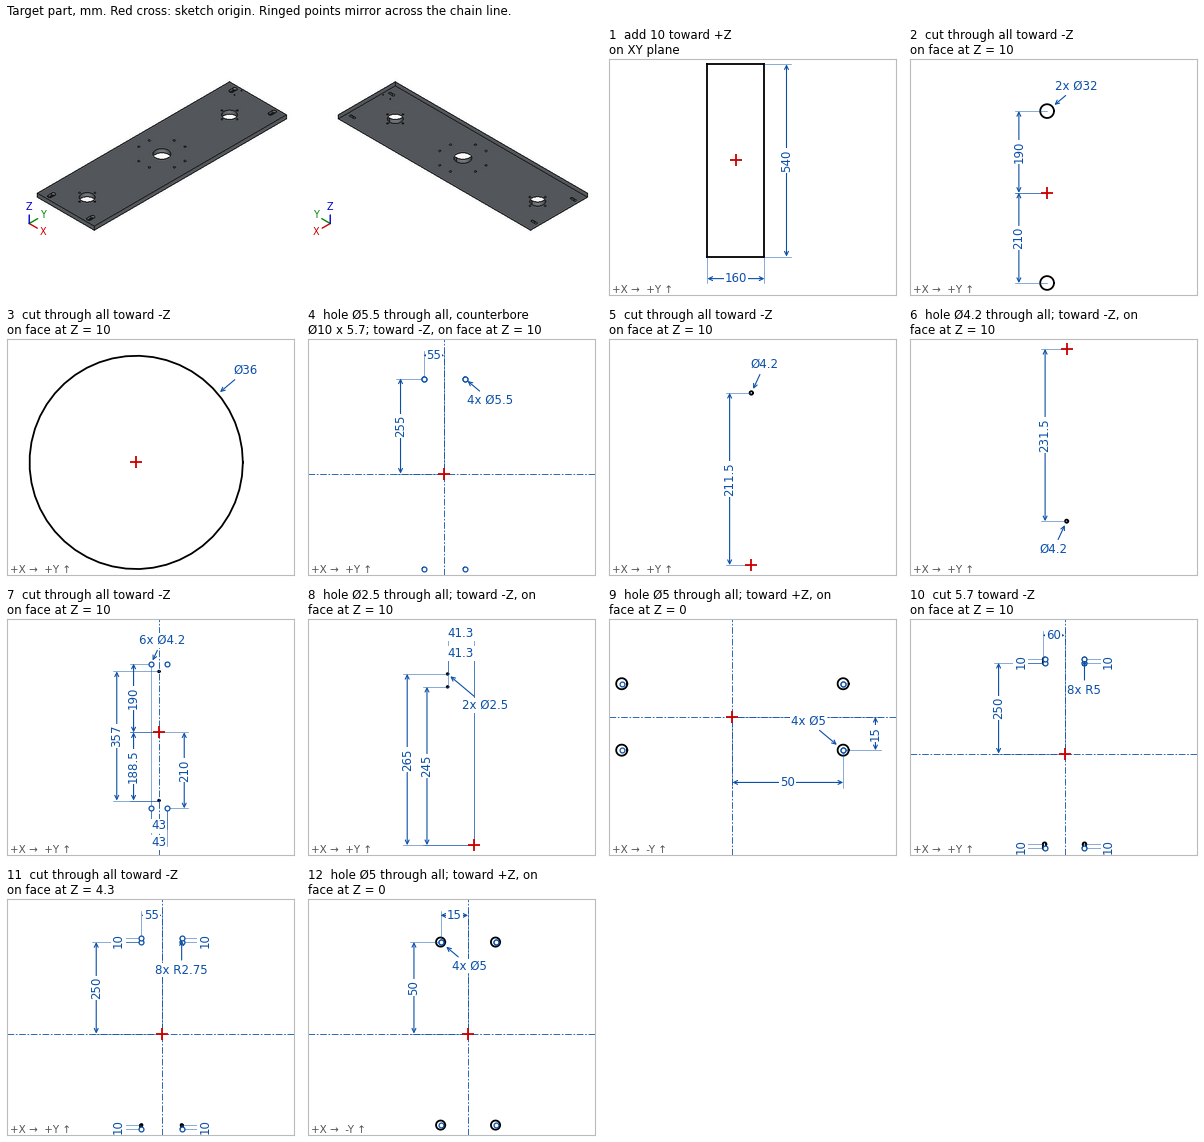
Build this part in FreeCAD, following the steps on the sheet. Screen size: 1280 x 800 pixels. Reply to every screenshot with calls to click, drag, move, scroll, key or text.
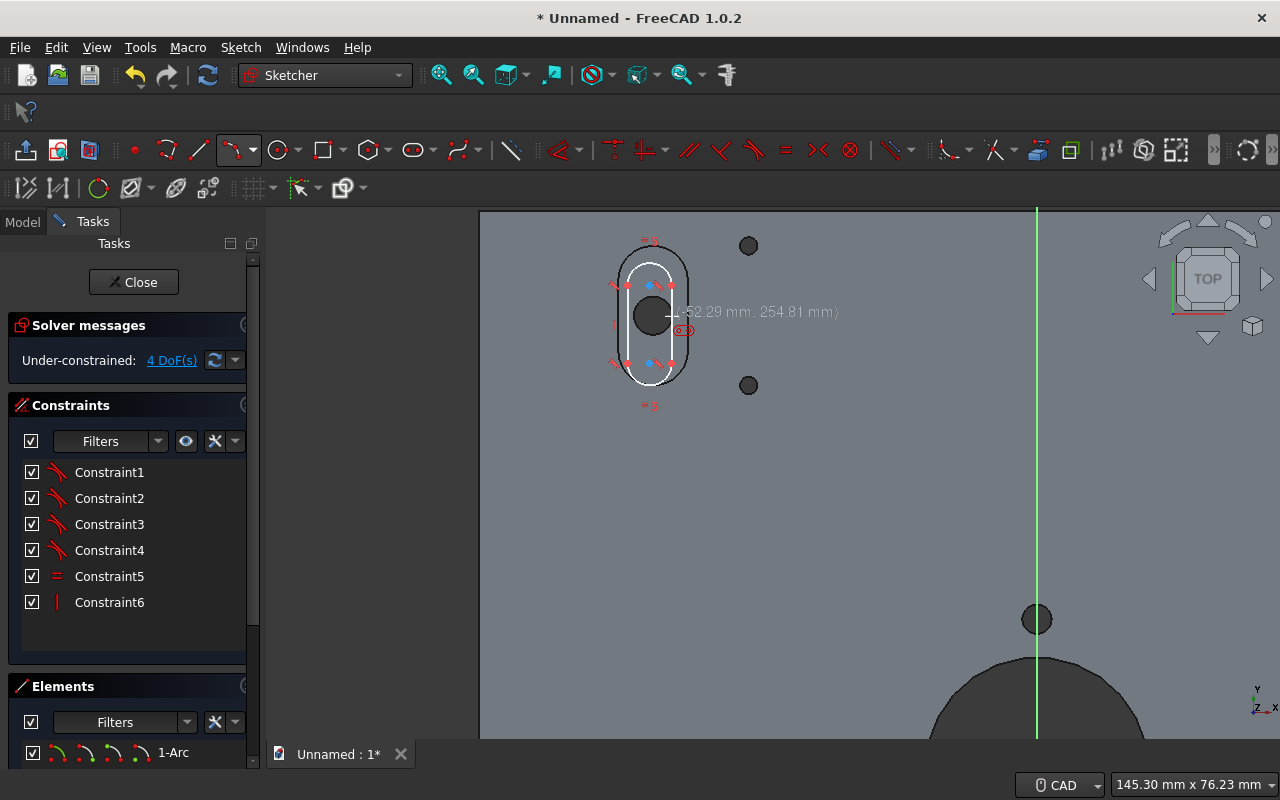
scroll(671, 311, down, 12)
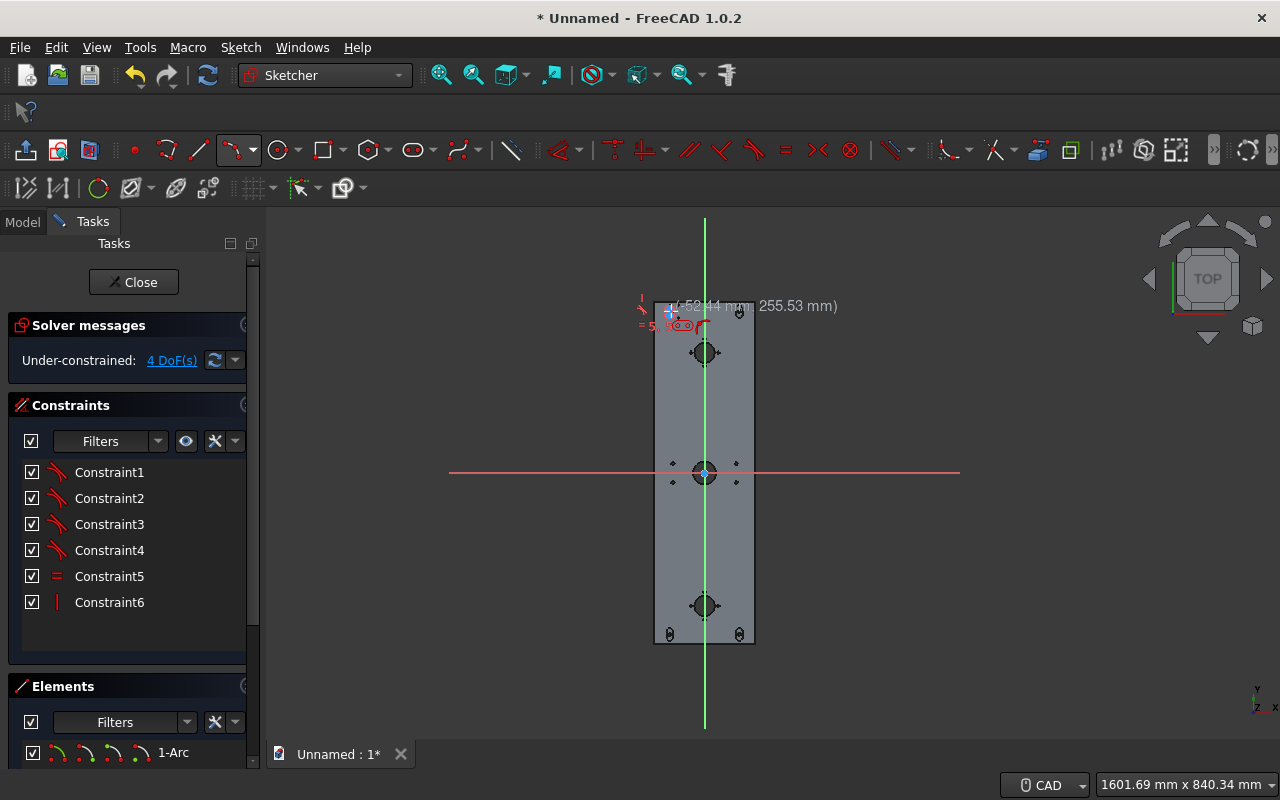
scroll(739, 315, up, 13)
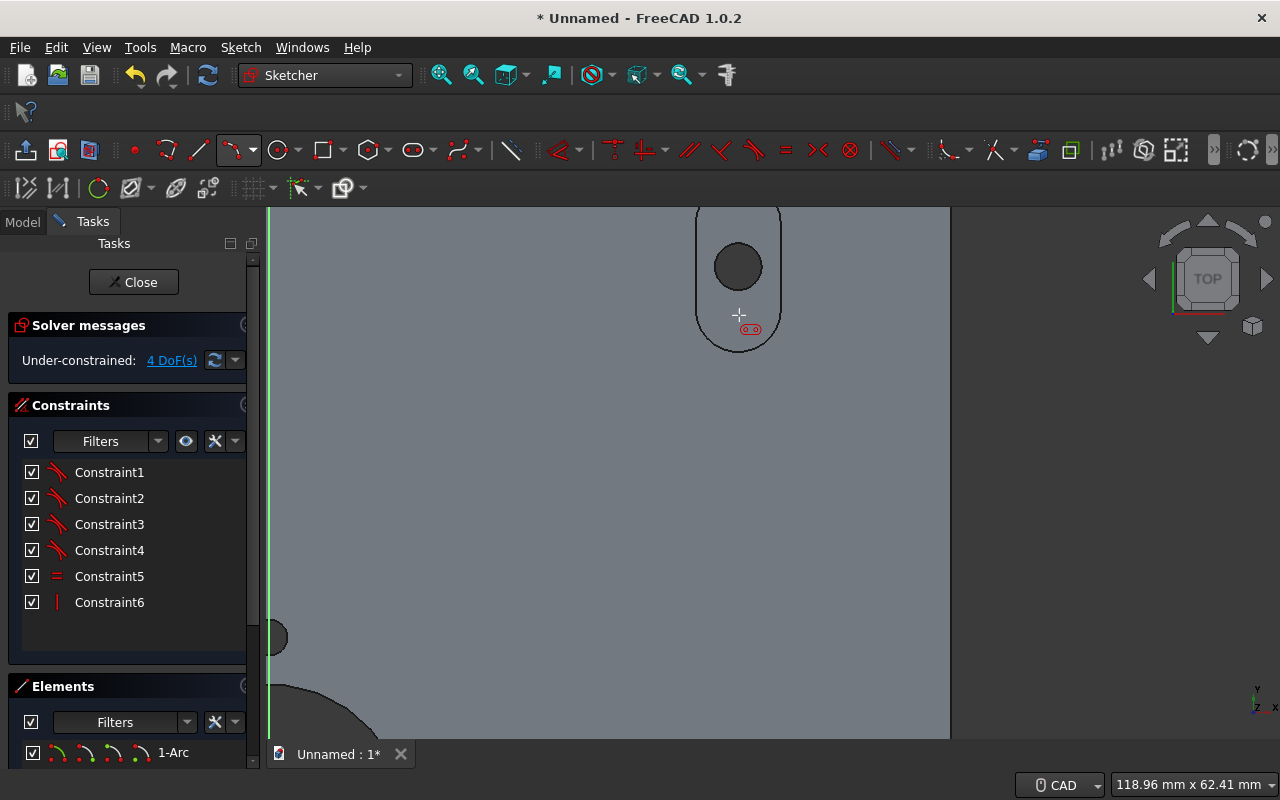
scroll(739, 315, down, 13)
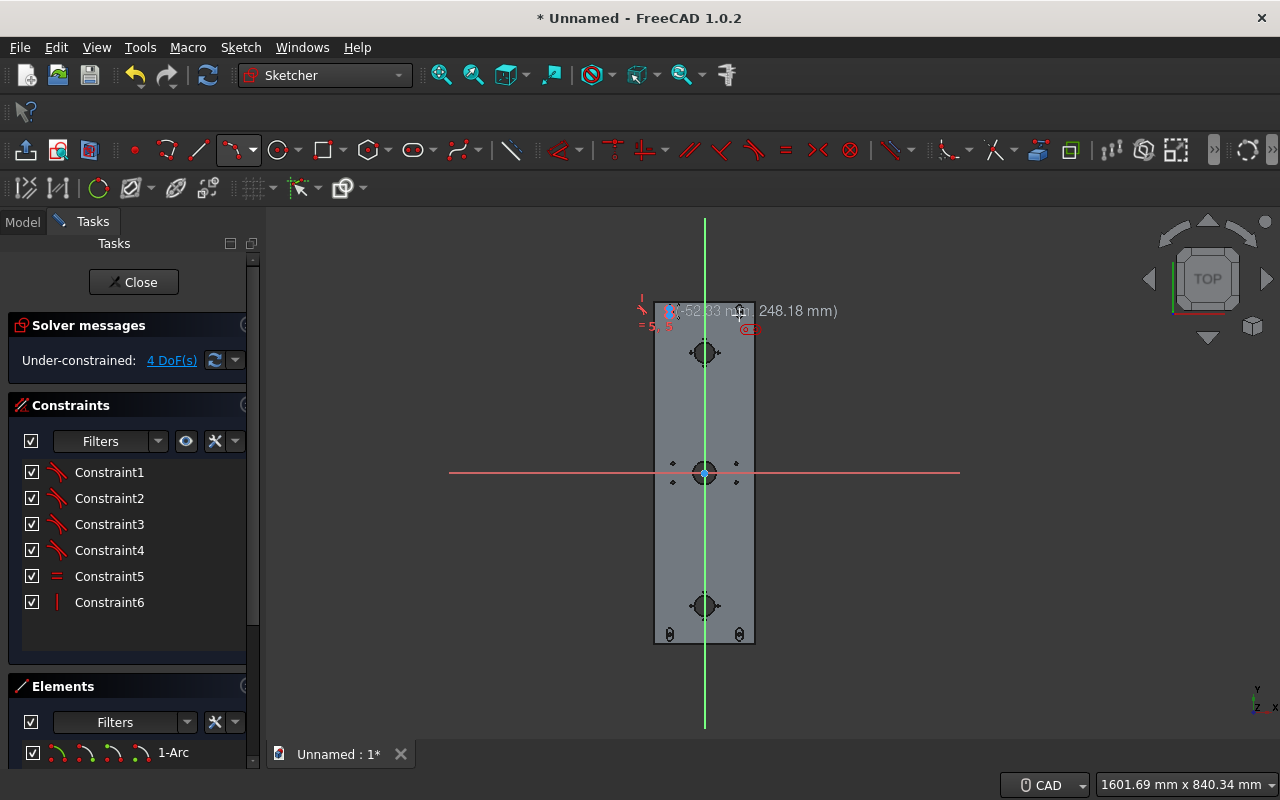
click(739, 315)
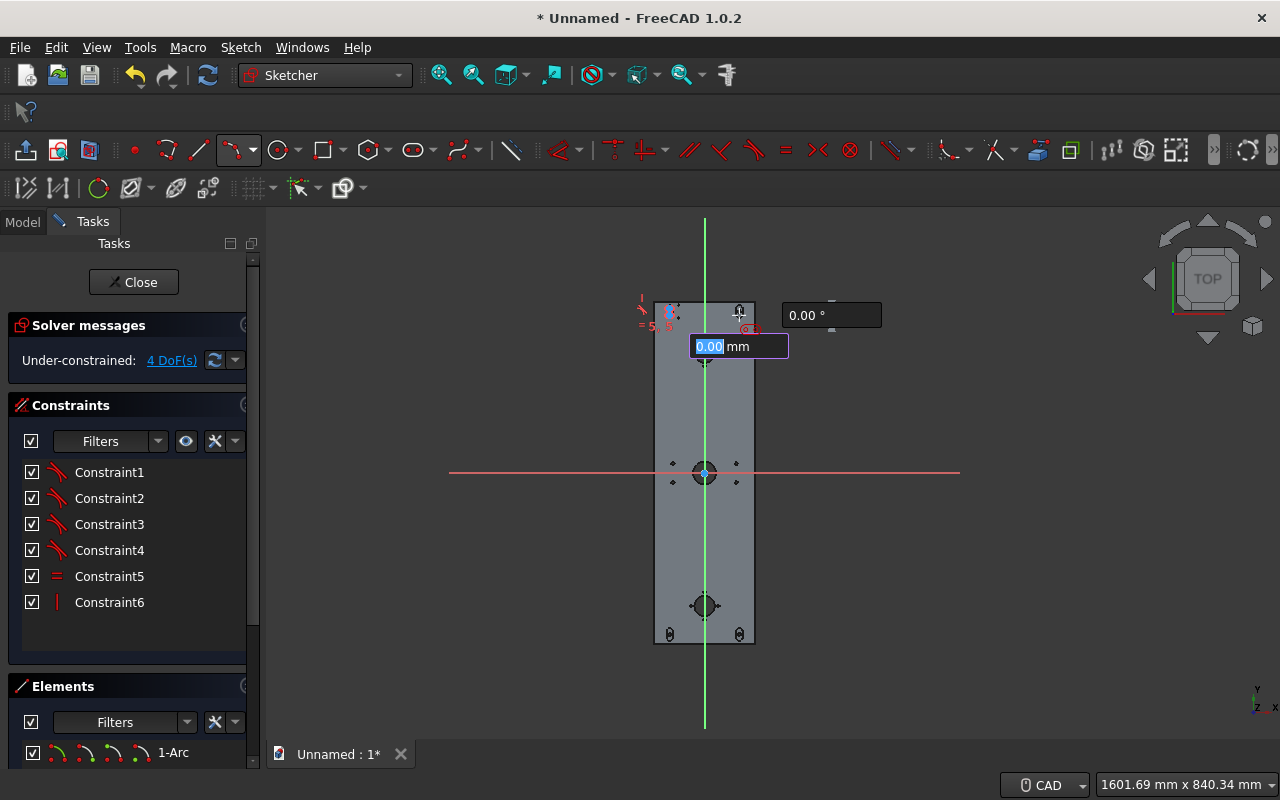
scroll(739, 308, up, 5)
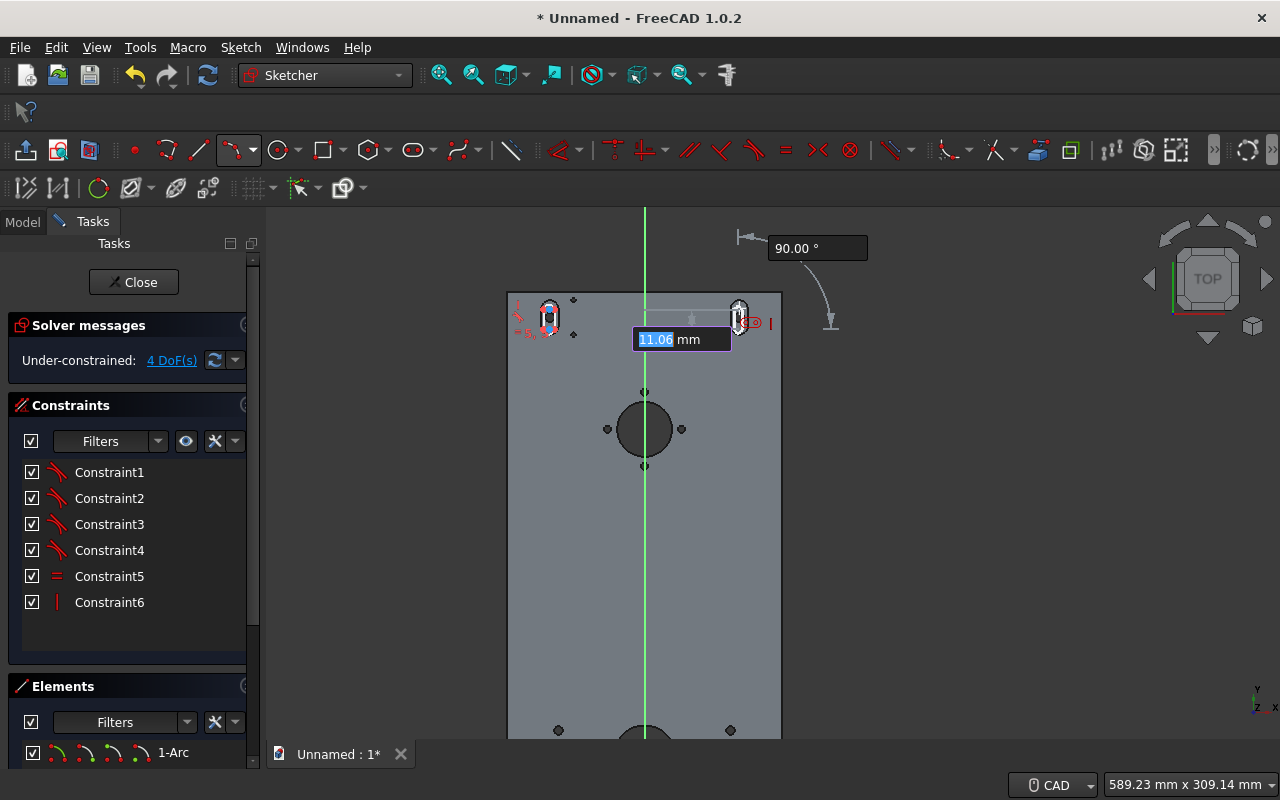
click(738, 309)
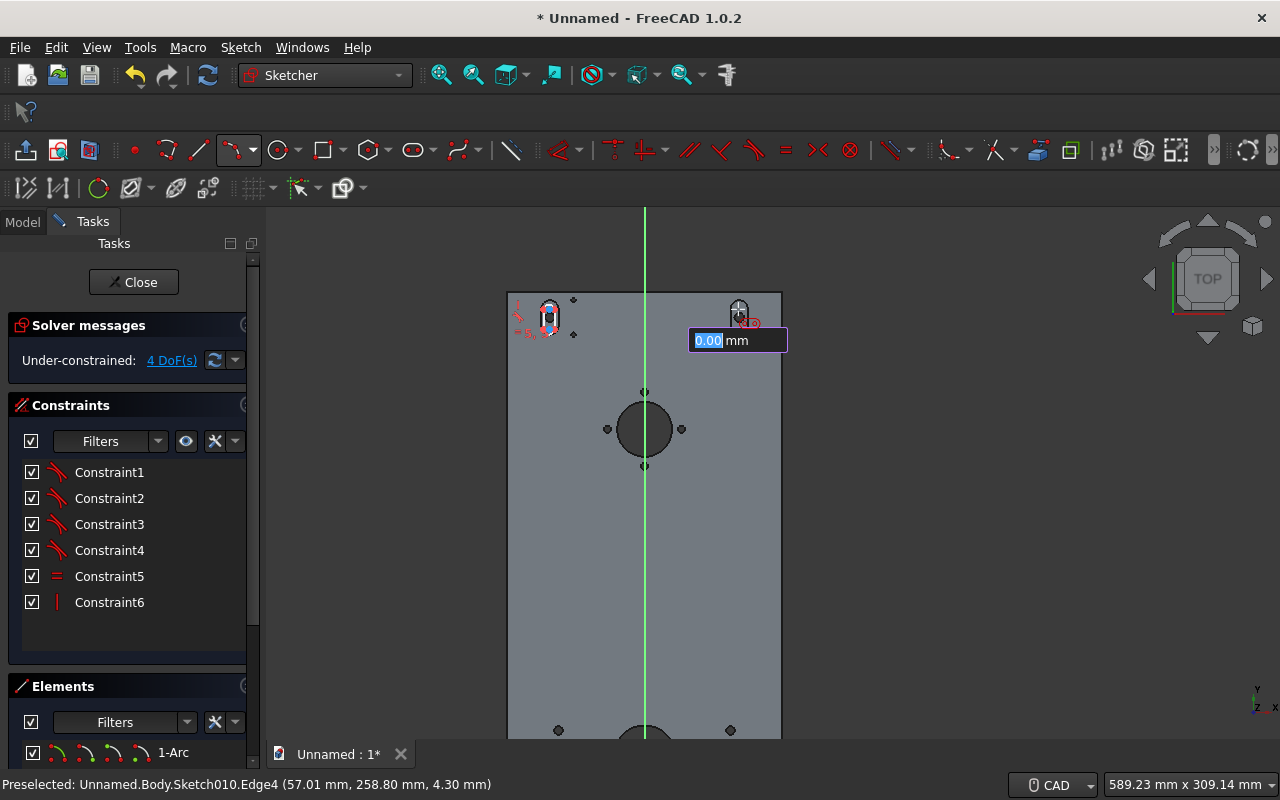
scroll(744, 317, up, 7)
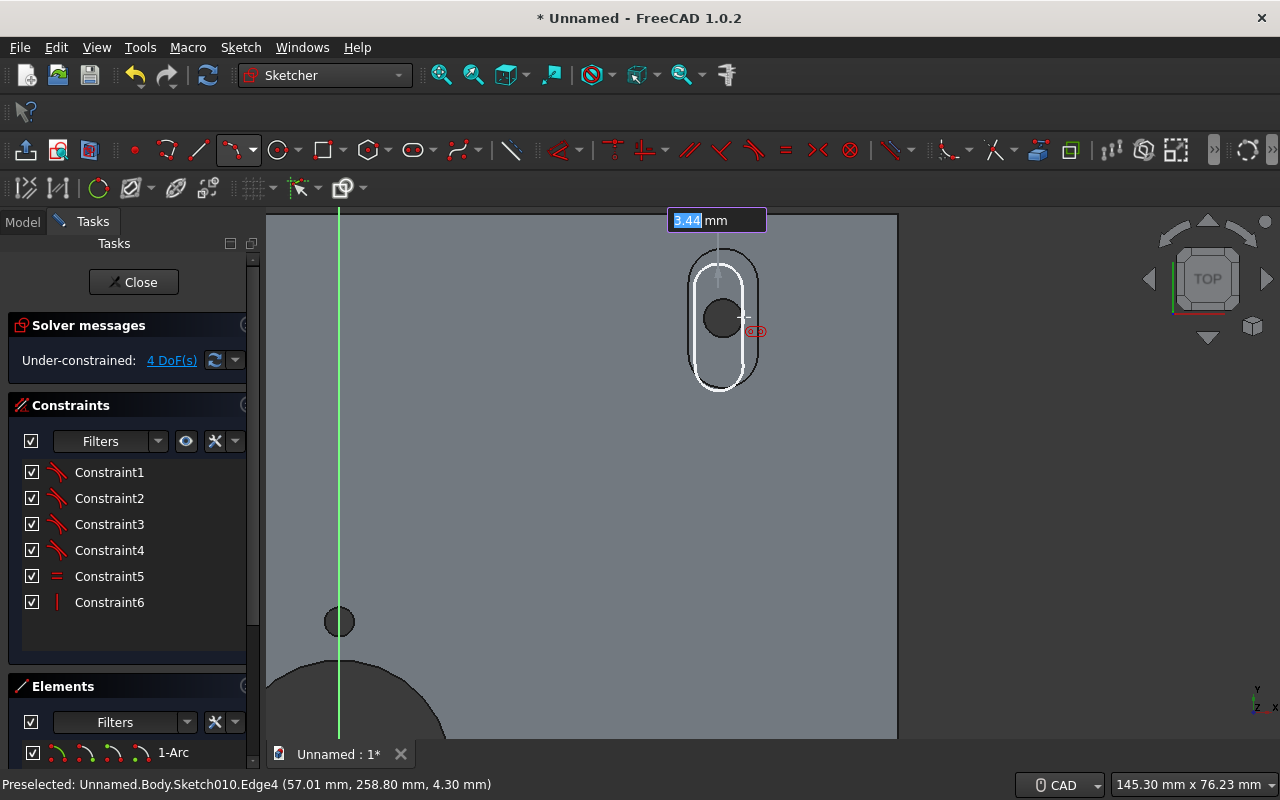
click(742, 318)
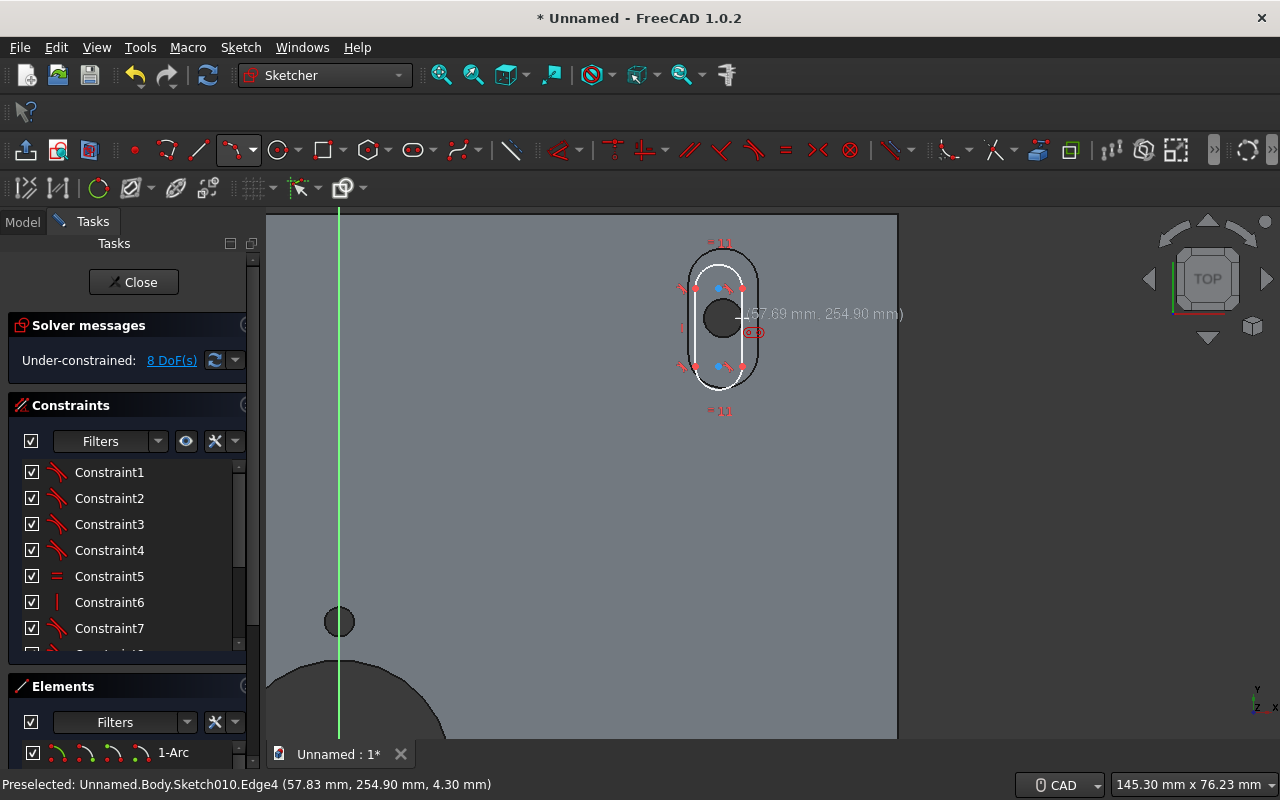
scroll(741, 311, down, 12)